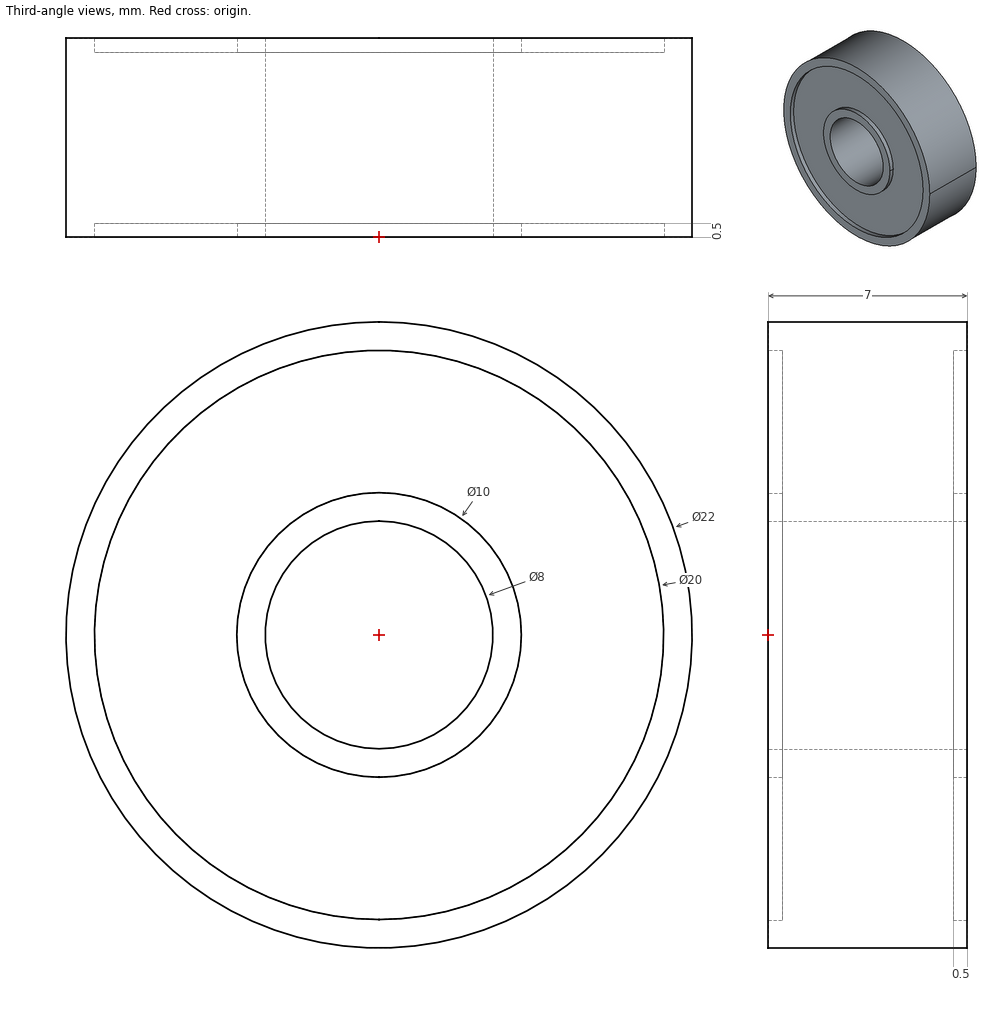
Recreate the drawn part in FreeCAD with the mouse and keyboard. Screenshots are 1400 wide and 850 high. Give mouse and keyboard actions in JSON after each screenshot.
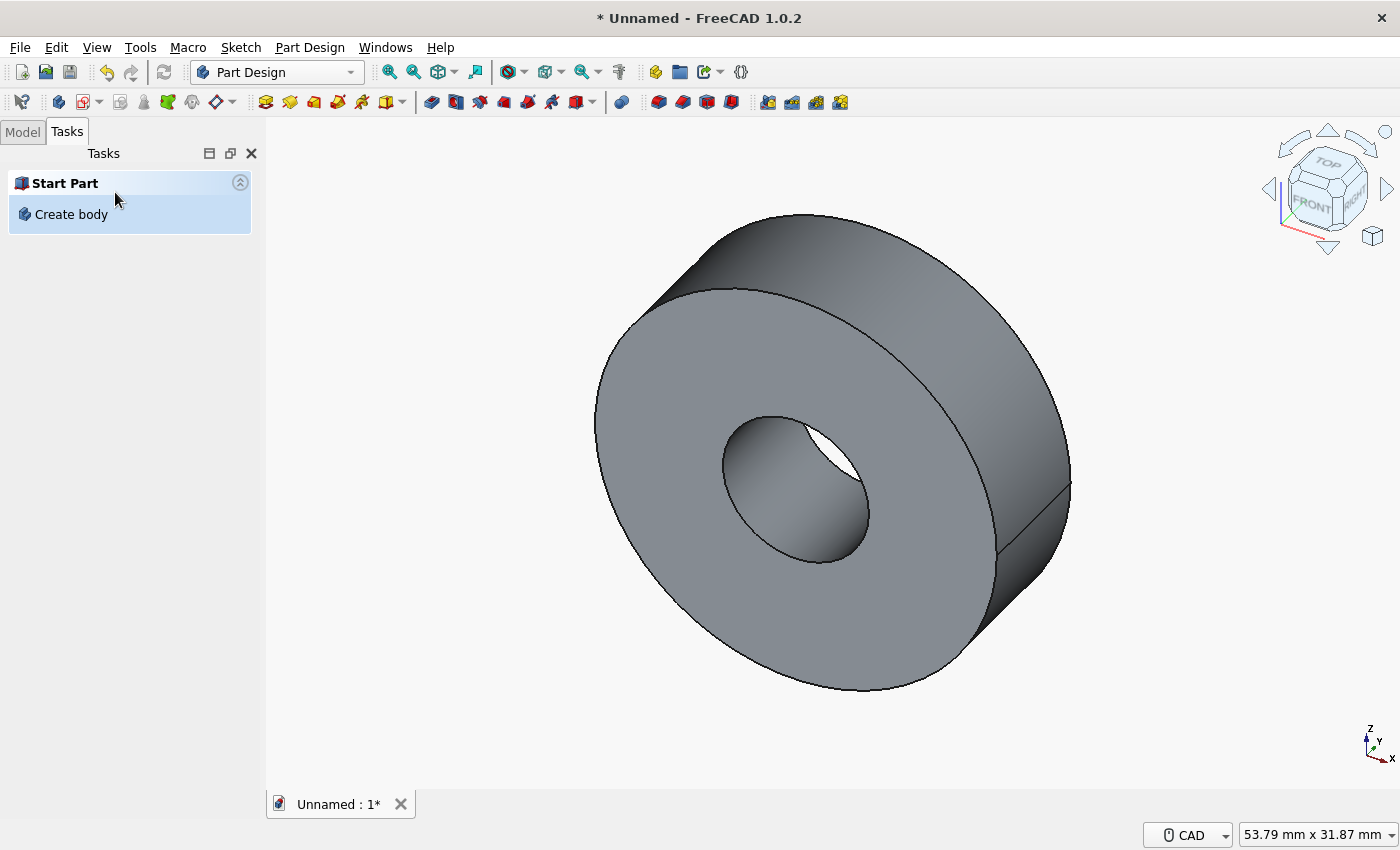
{"action": "left_click", "coordinate": [681, 505]}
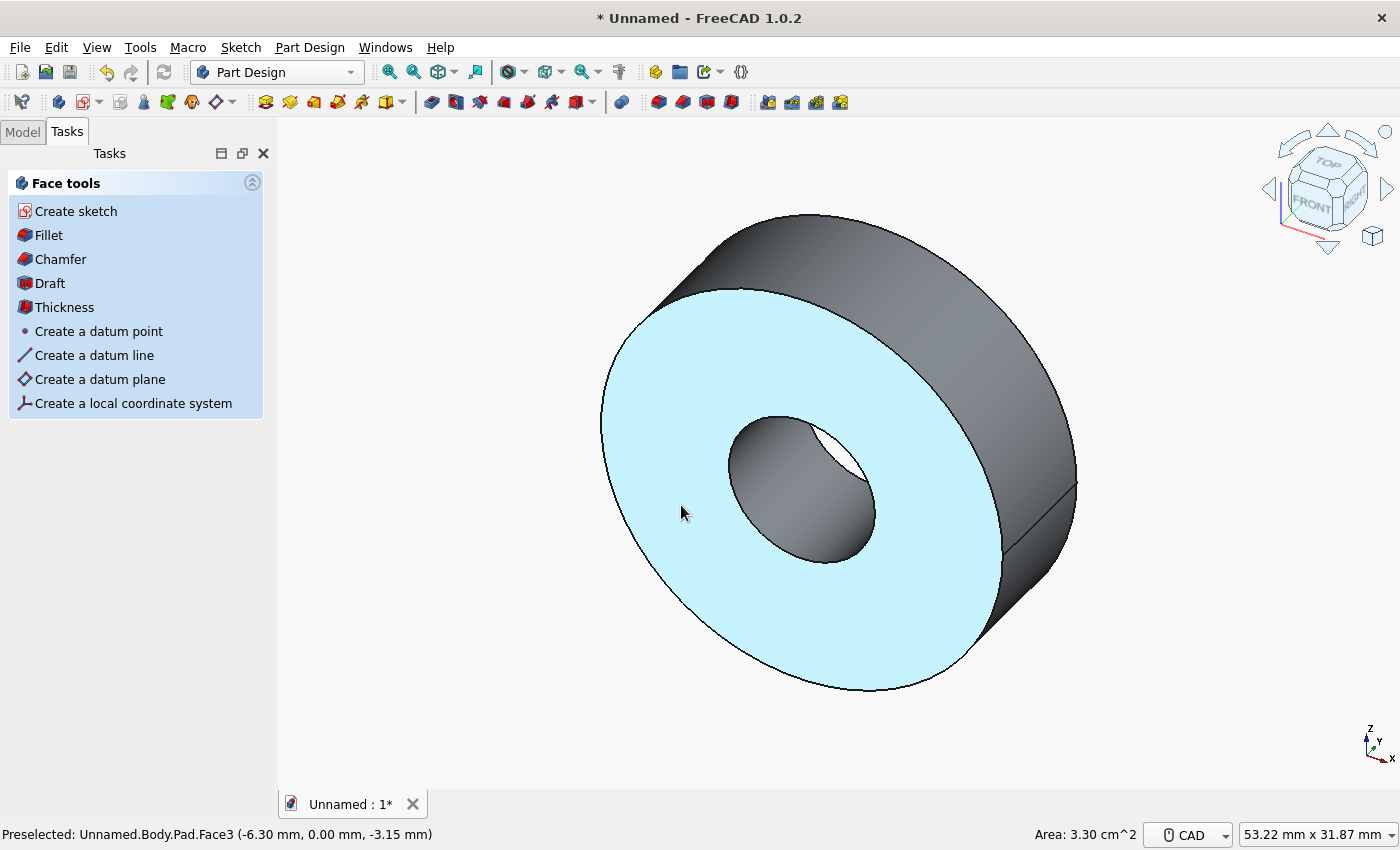
{"action": "left_click", "coordinate": [84, 102]}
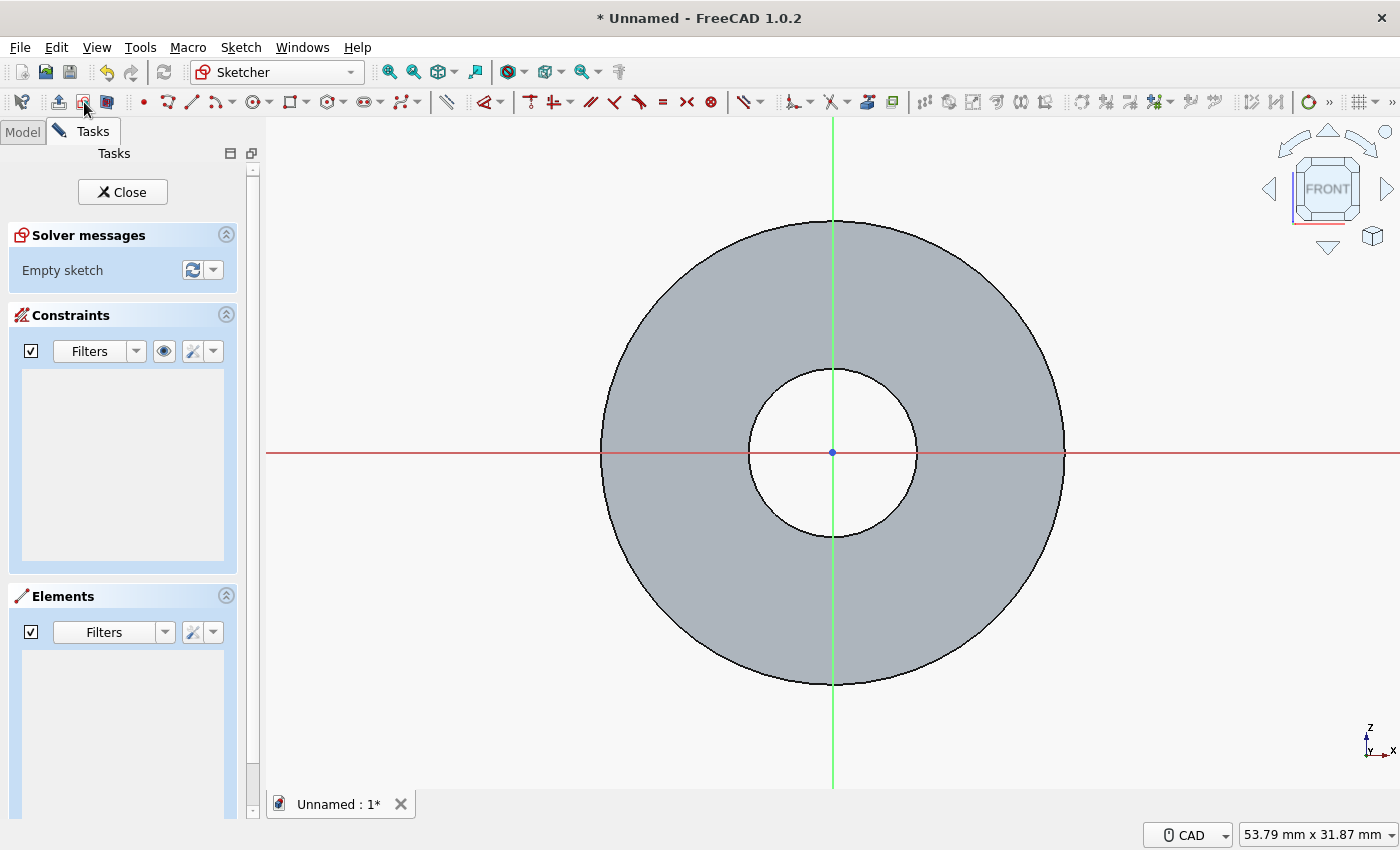
{"action": "key", "text": "g c"}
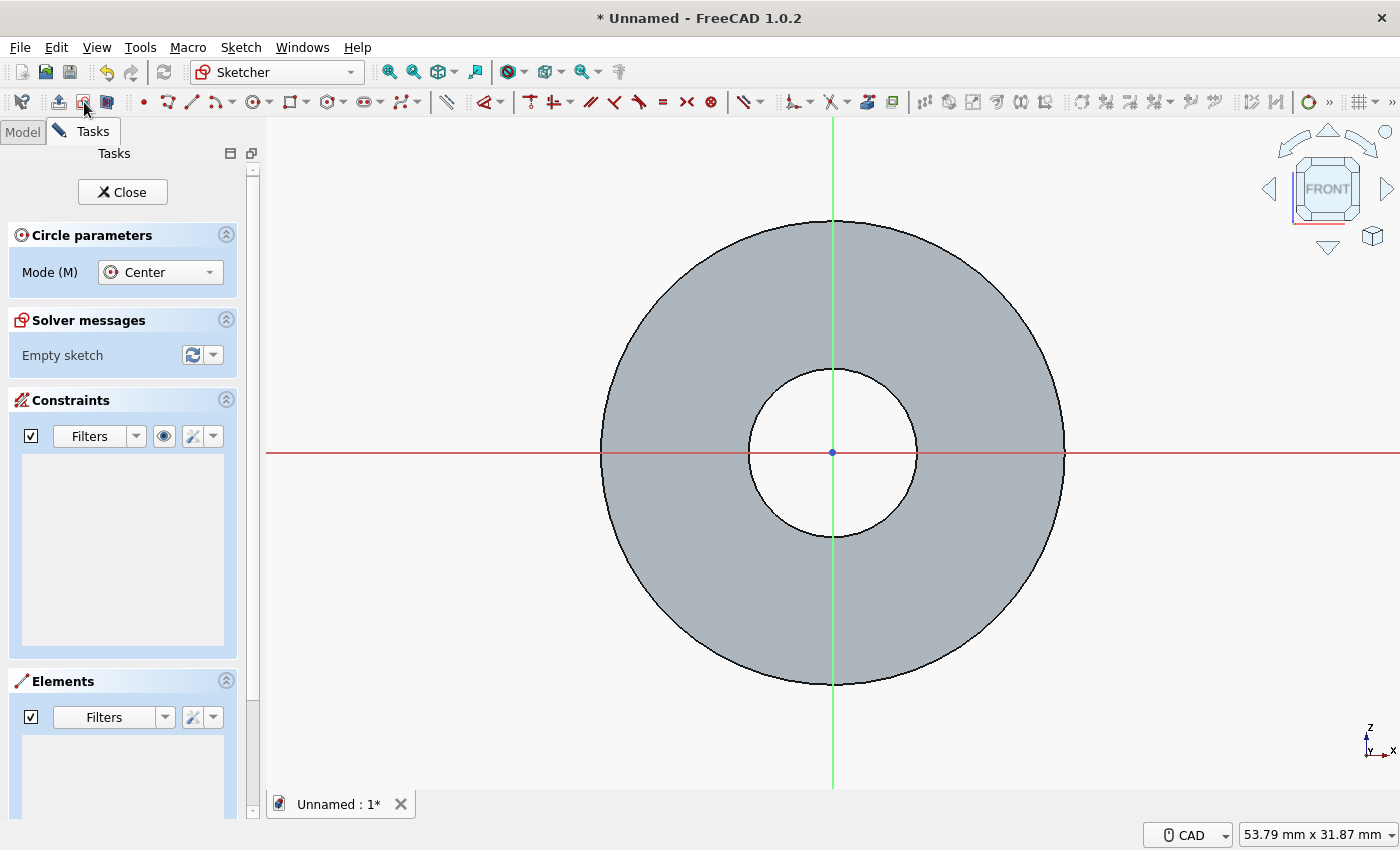
{"action": "left_click", "coordinate": [833, 453]}
{"action": "mouse_move", "coordinate": [982, 304]}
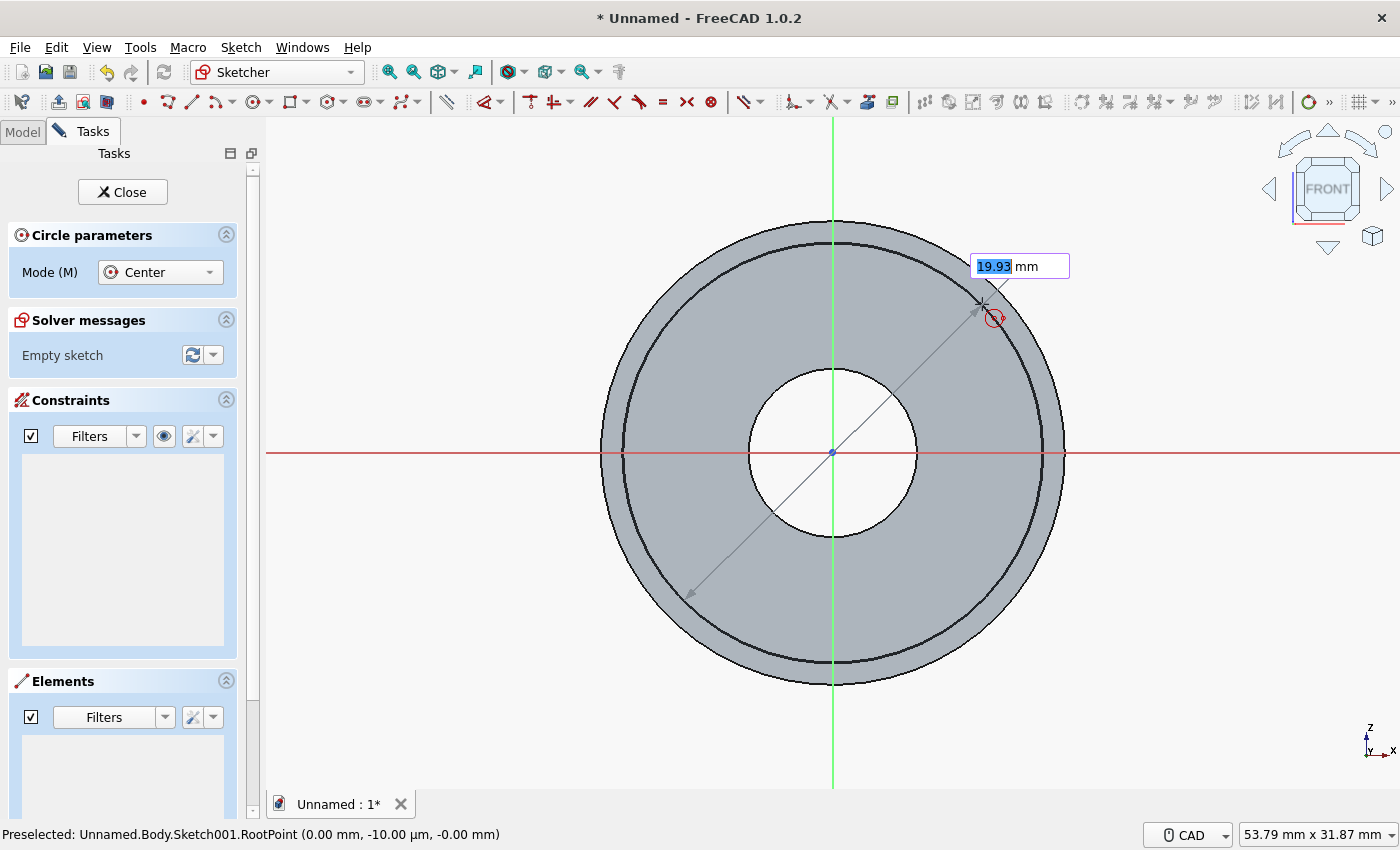
{"action": "type", "text": "20"}
{"action": "key", "text": "Return"}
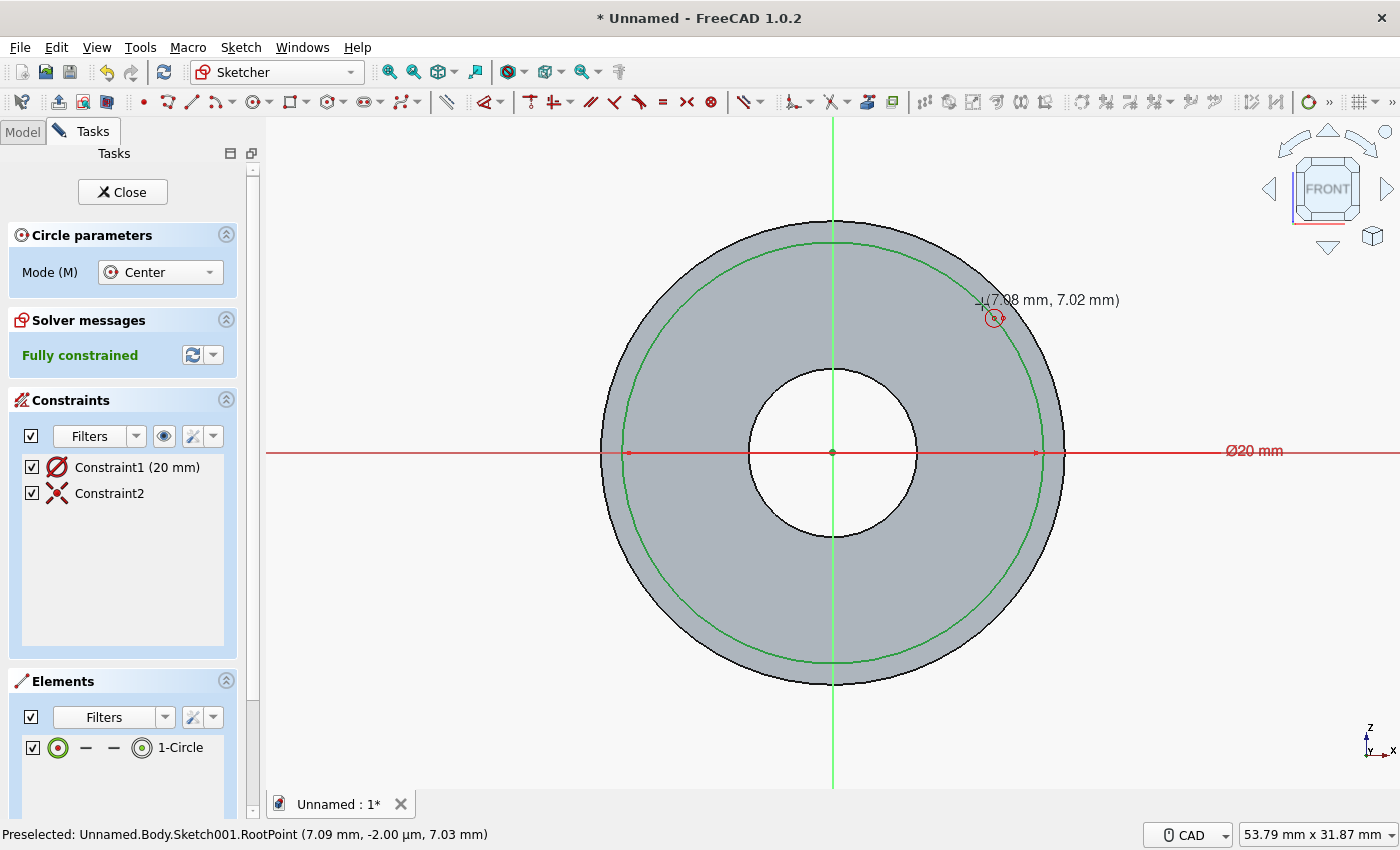
{"action": "left_click", "coordinate": [833, 453]}
{"action": "mouse_move", "coordinate": [907, 378]}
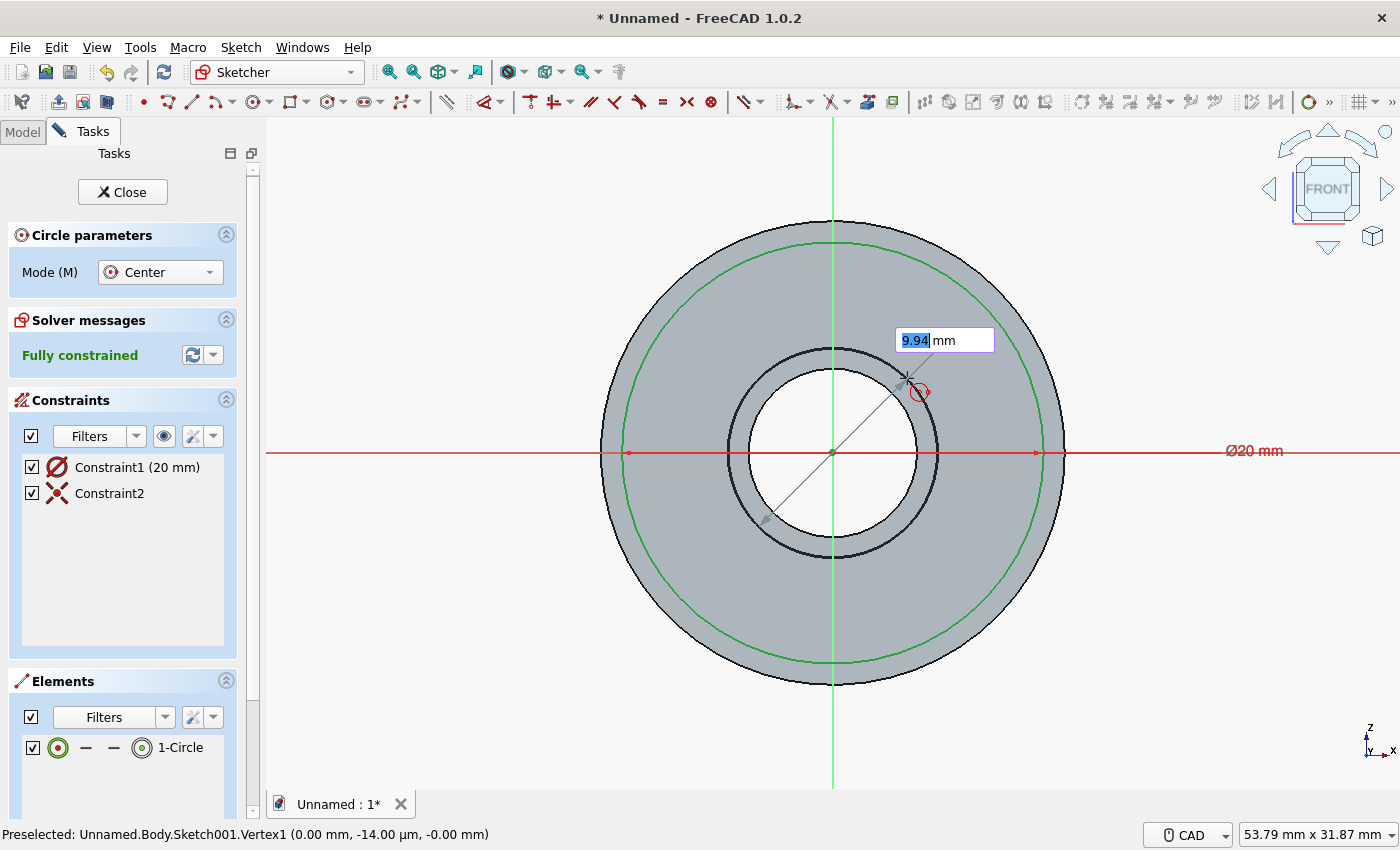
{"action": "type", "text": "10"}
{"action": "key", "text": "Return"}
{"action": "key", "text": "Escape"}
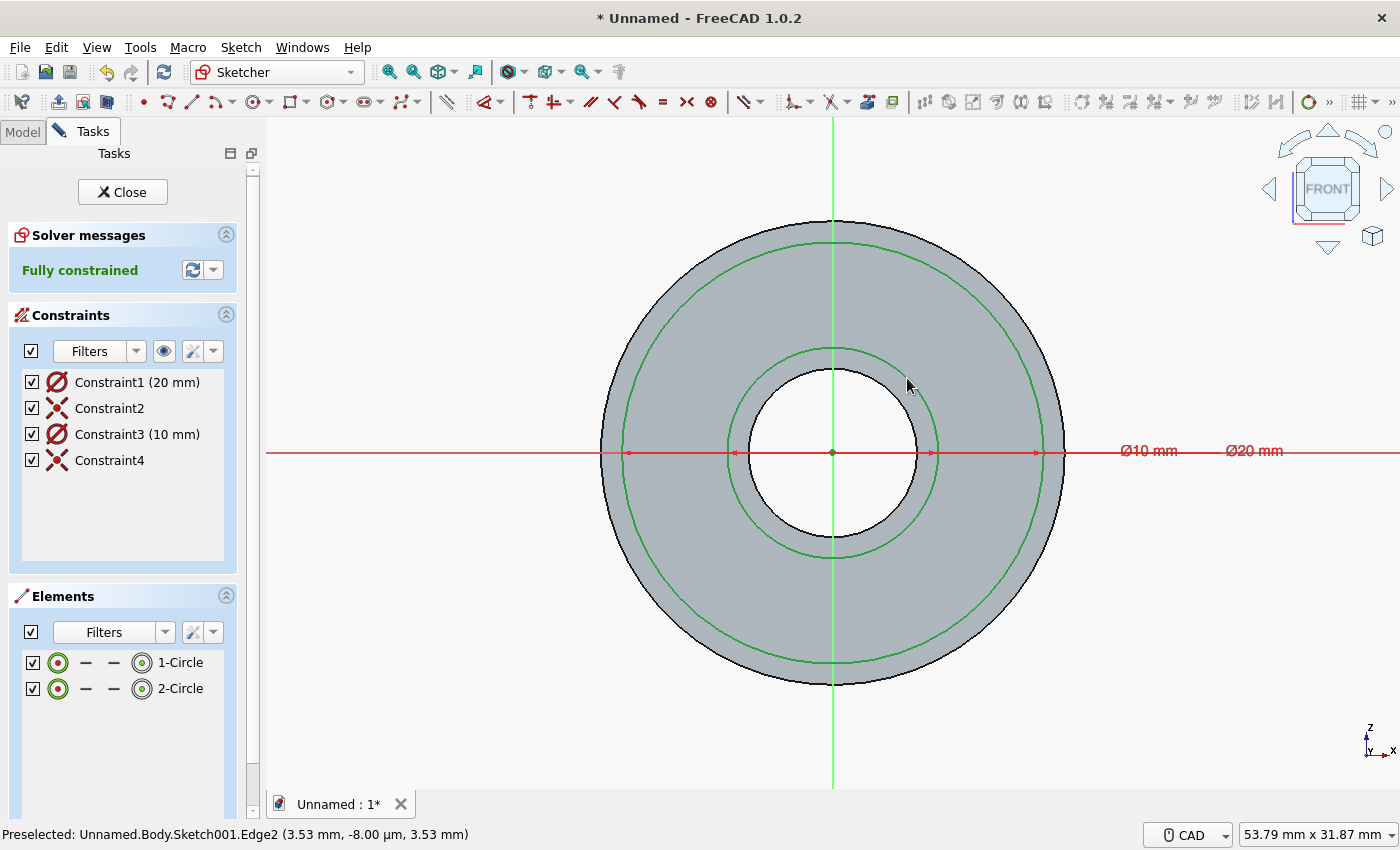
{"action": "left_click", "coordinate": [123, 192]}